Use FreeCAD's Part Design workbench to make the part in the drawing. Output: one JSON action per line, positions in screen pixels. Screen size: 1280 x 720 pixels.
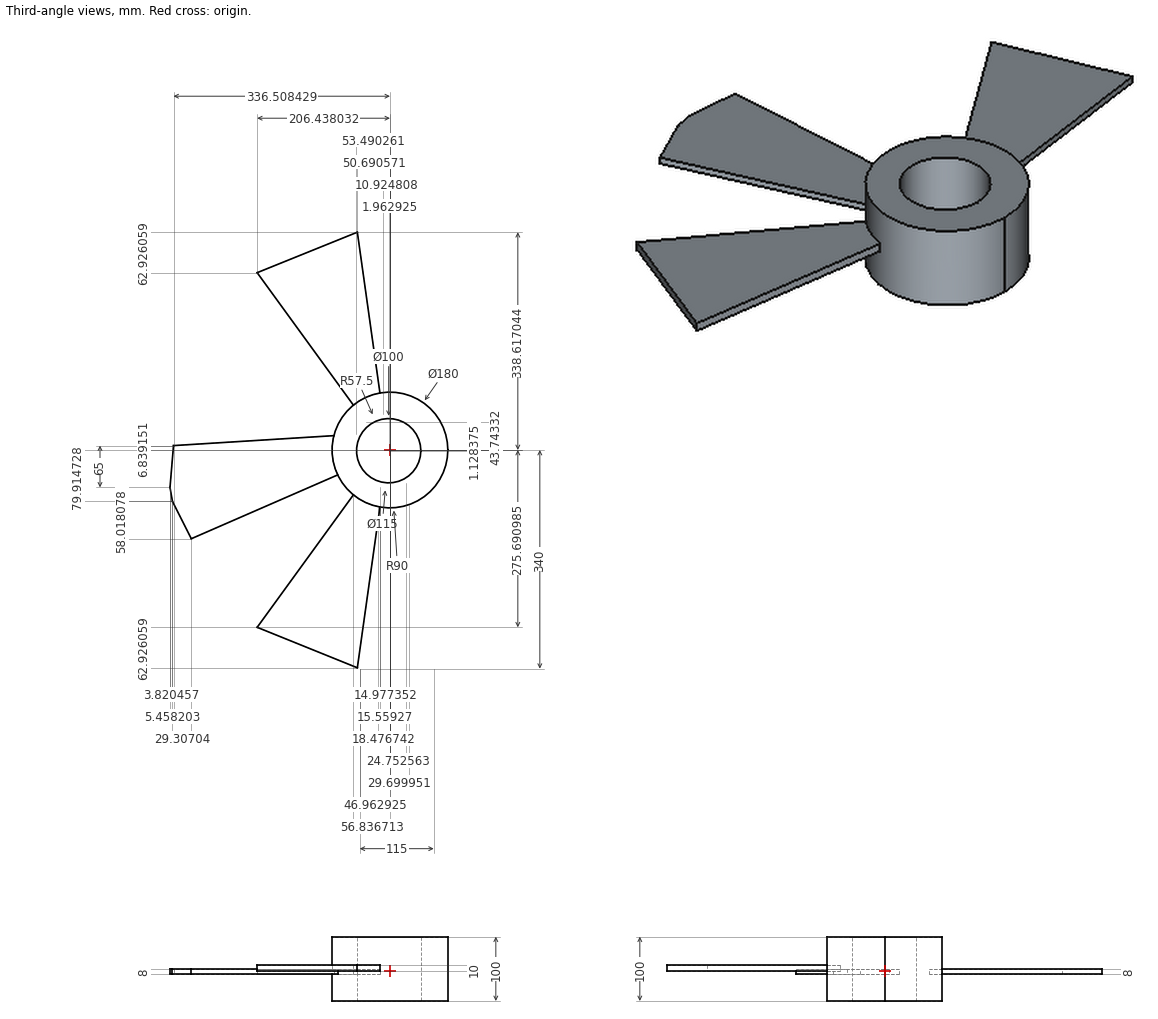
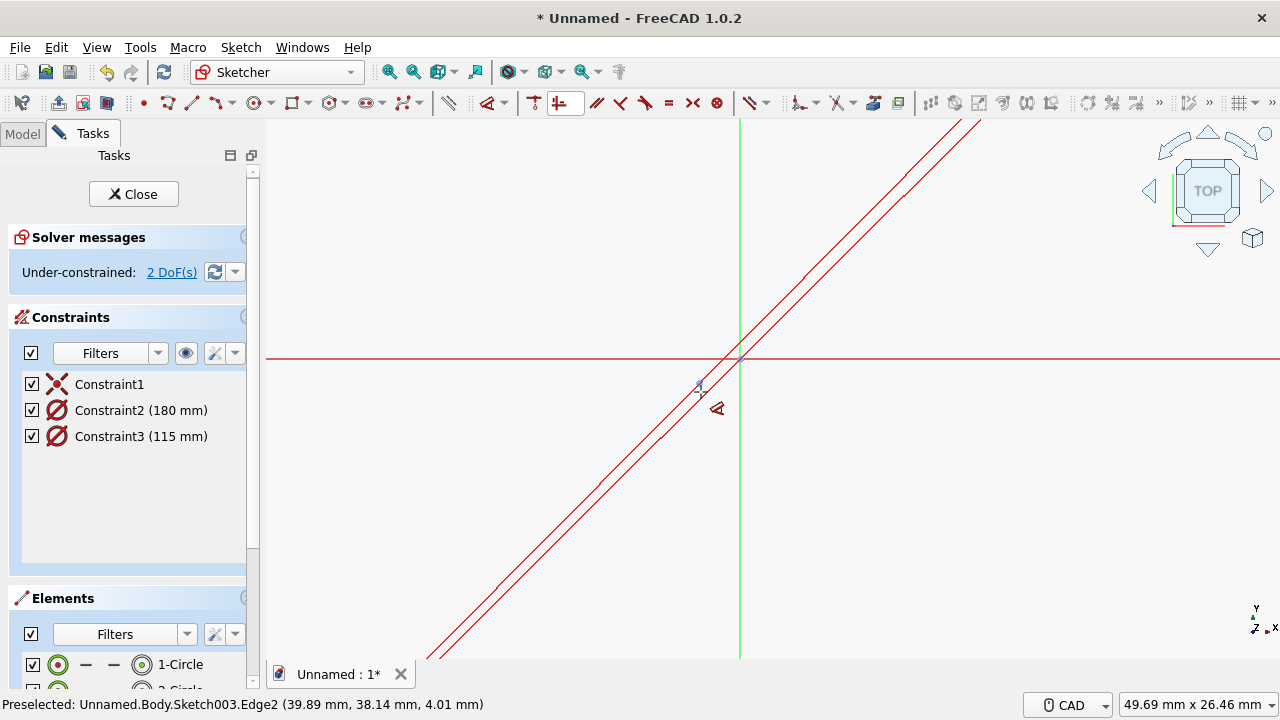
{"action": "left_click", "coordinate": [700, 383]}
{"action": "left_click", "coordinate": [720, 417]}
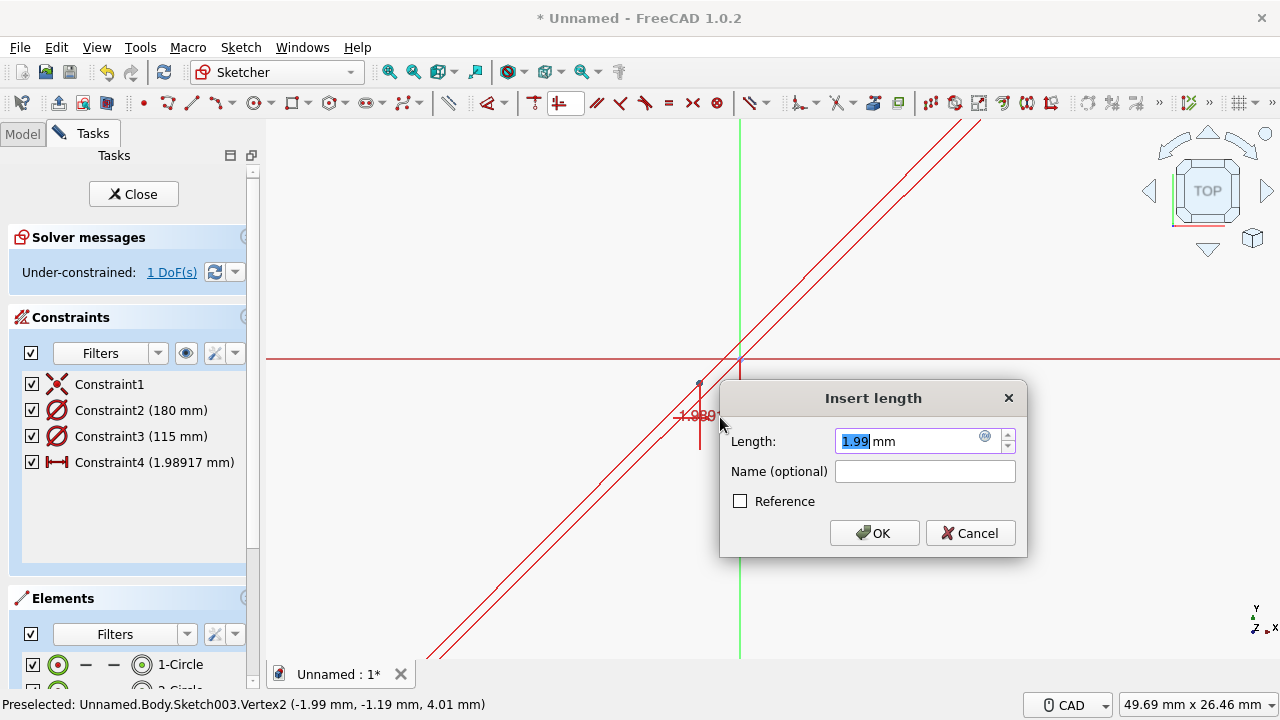
{"action": "type", "text": "1.962925"}
{"action": "key", "text": "Return"}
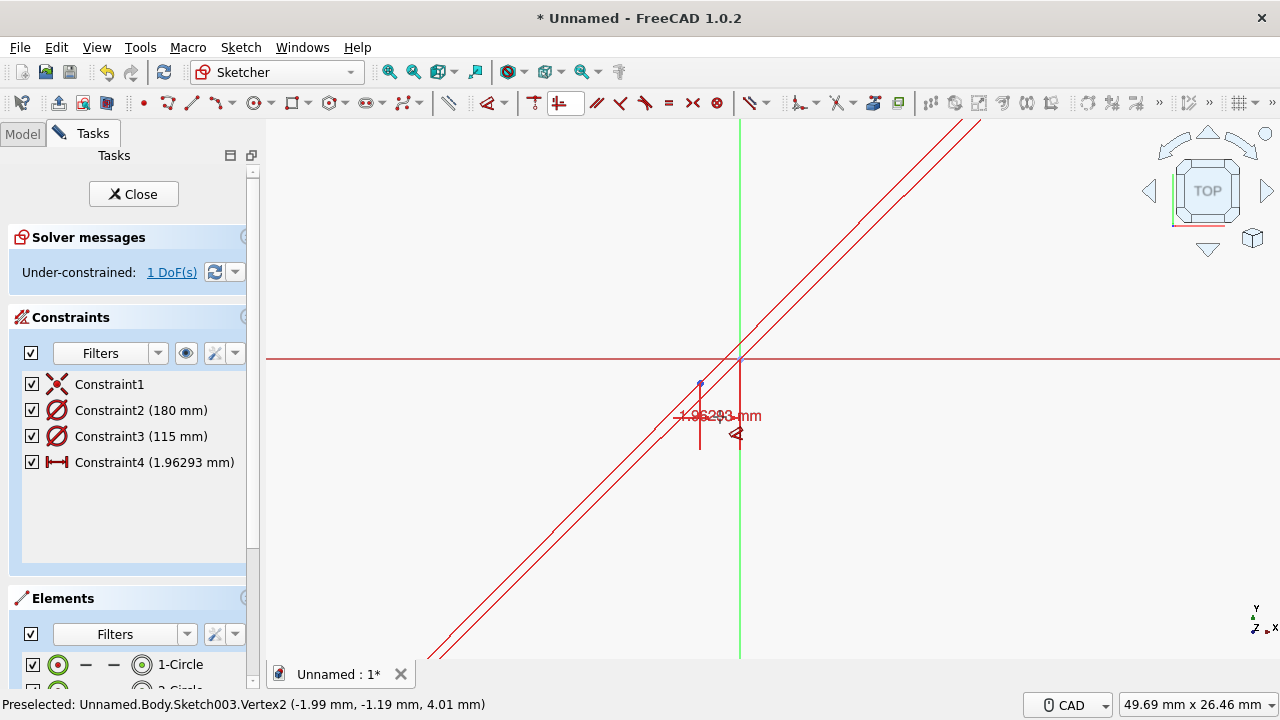
{"action": "scroll", "coordinate": [700, 383], "scroll_direction": "up", "scroll_amount": 3}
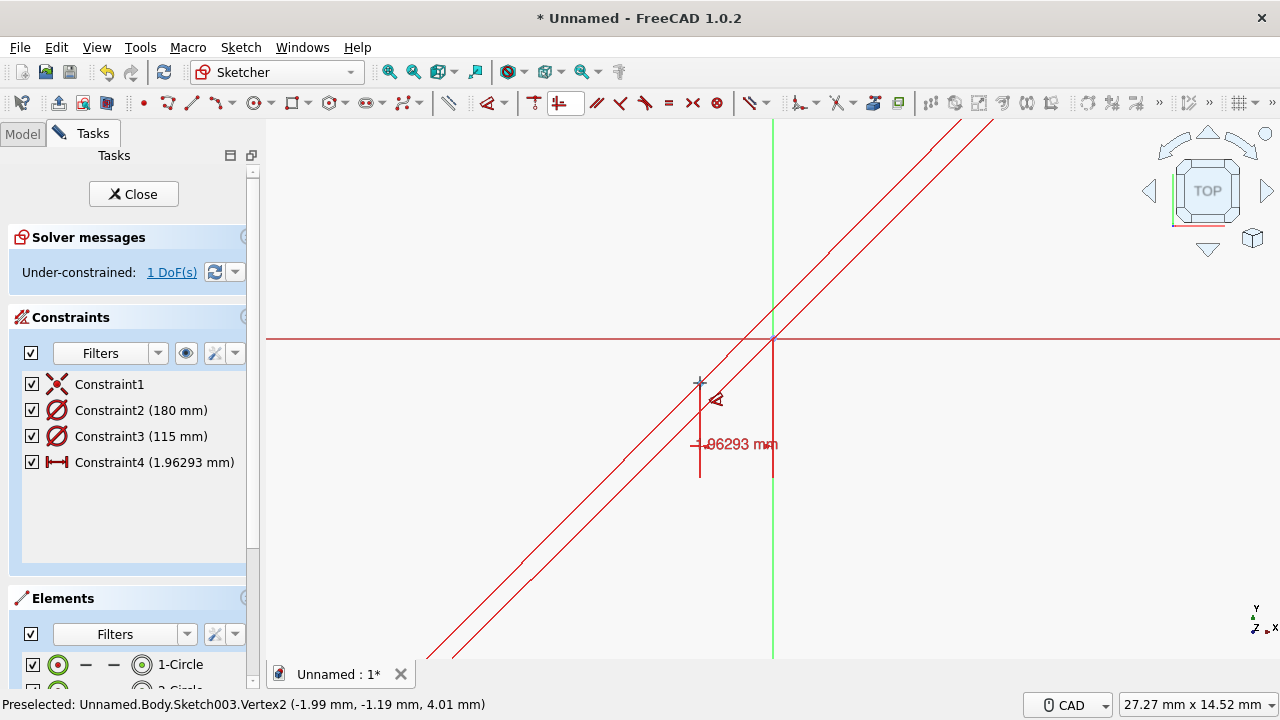
{"action": "left_click", "coordinate": [700, 383]}
{"action": "left_click", "coordinate": [666, 361]}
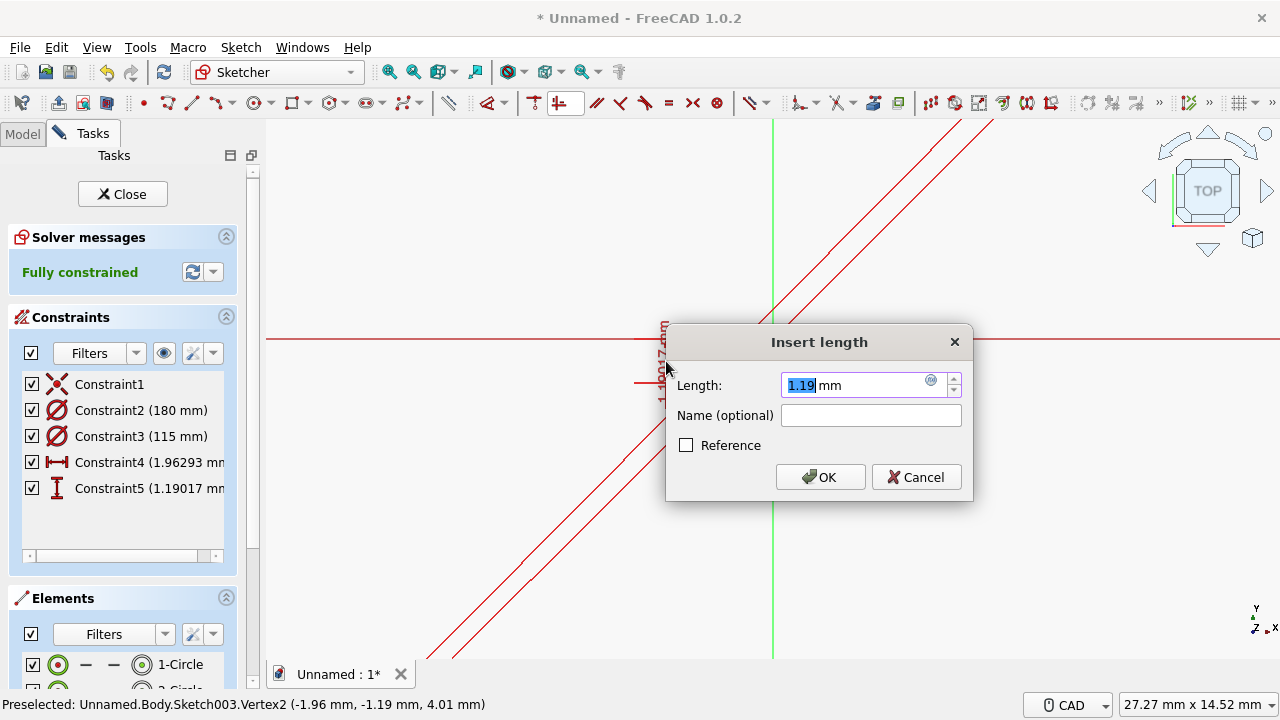
{"action": "type", "text": "1.128375"}
{"action": "key", "text": "Return"}
{"action": "key", "text": "Escape"}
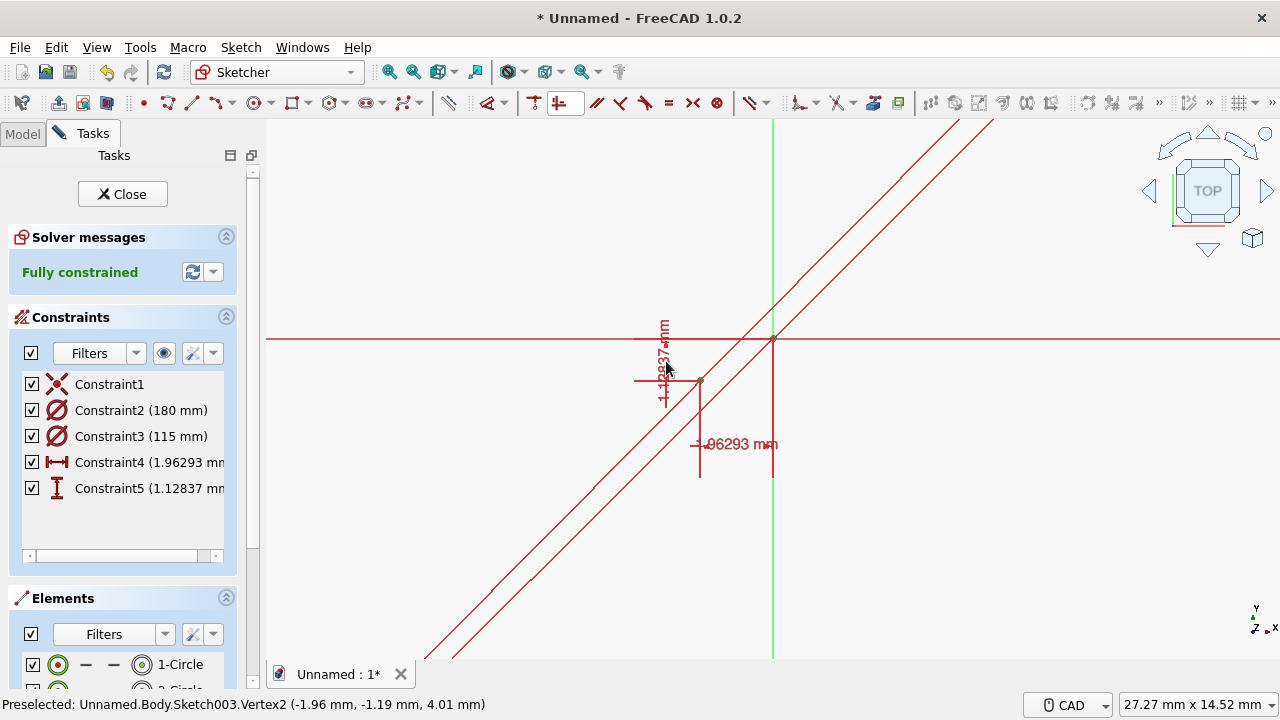
{"action": "left_click", "coordinate": [123, 194]}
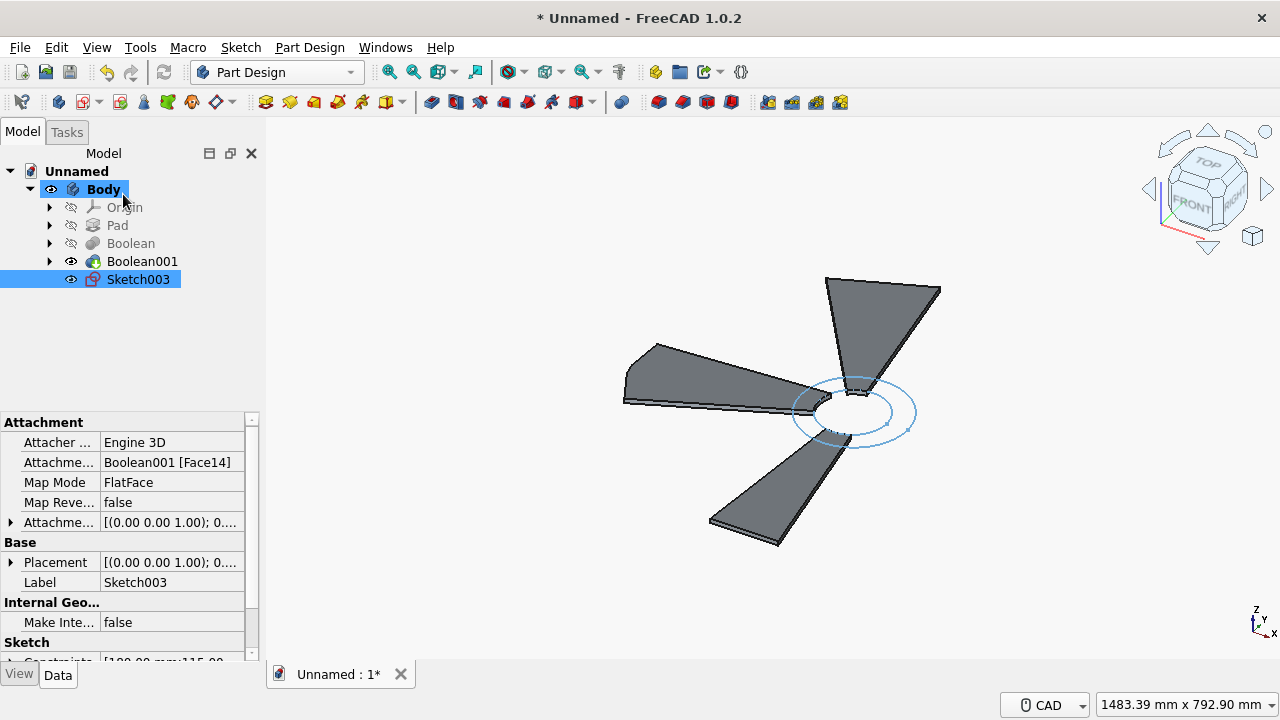
{"action": "left_click", "coordinate": [266, 102]}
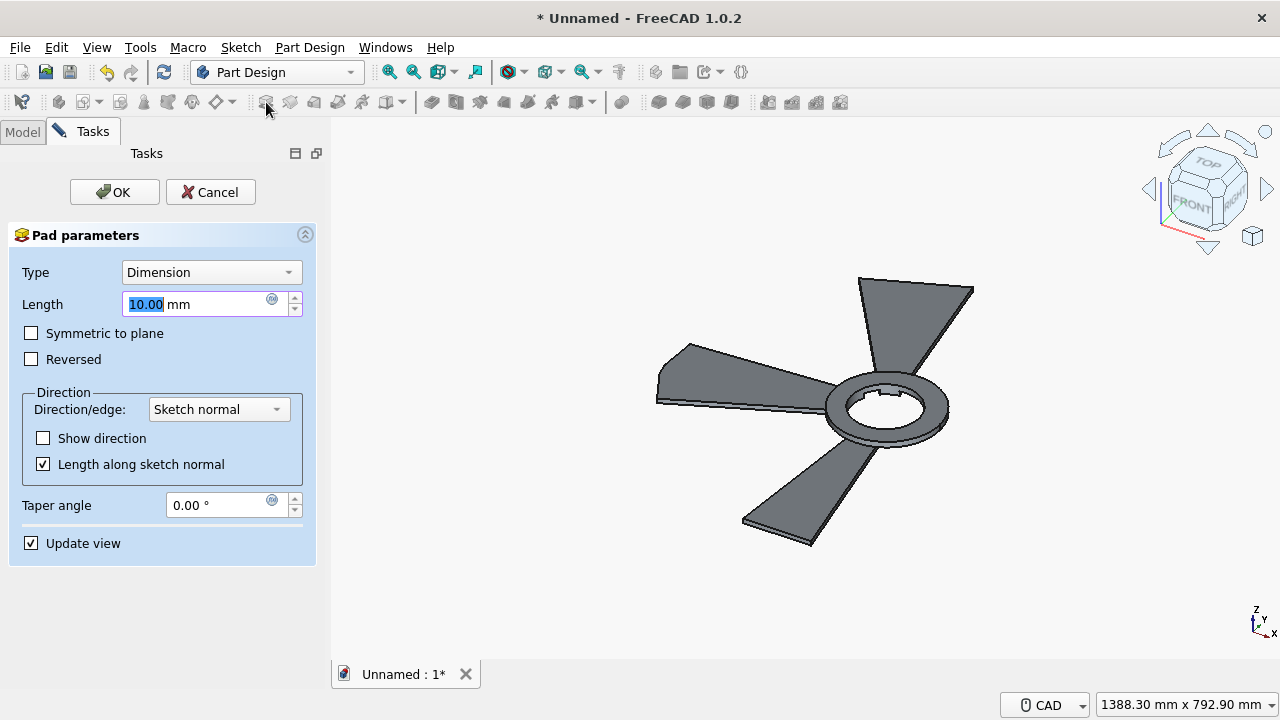
{"action": "type", "text": "100"}
{"action": "key", "text": "Tab"}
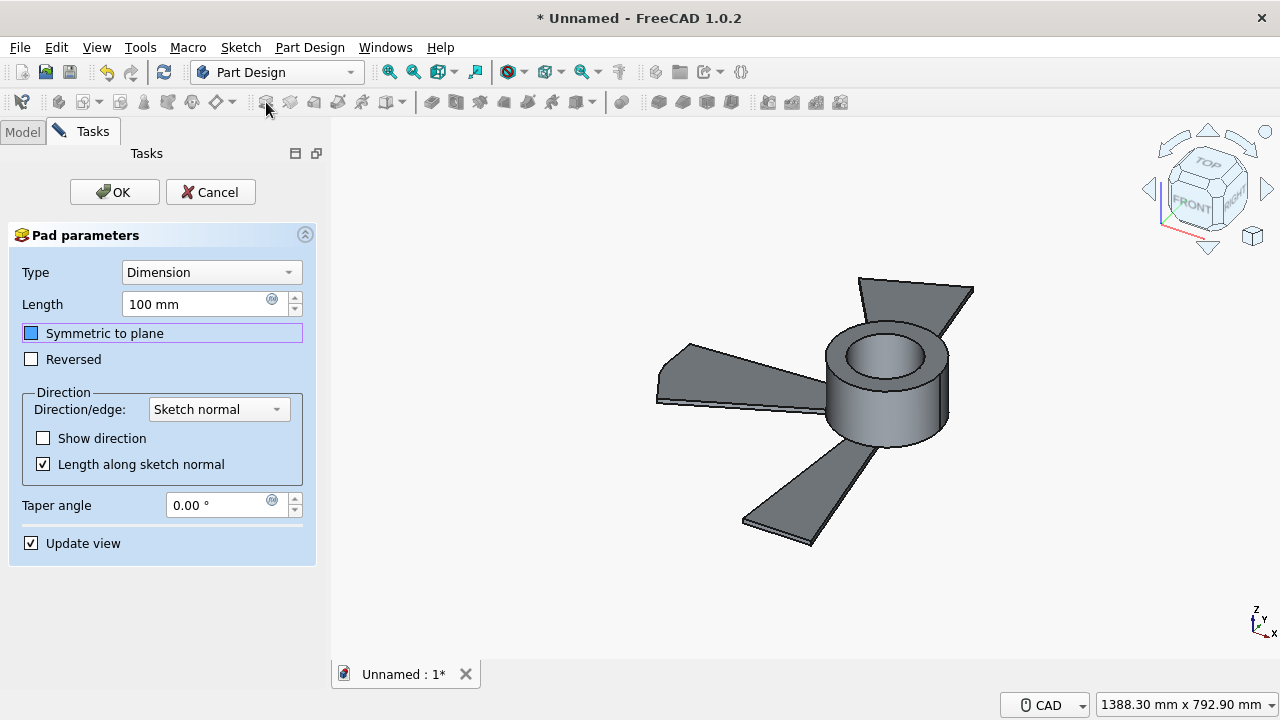
{"action": "left_click", "coordinate": [30, 333]}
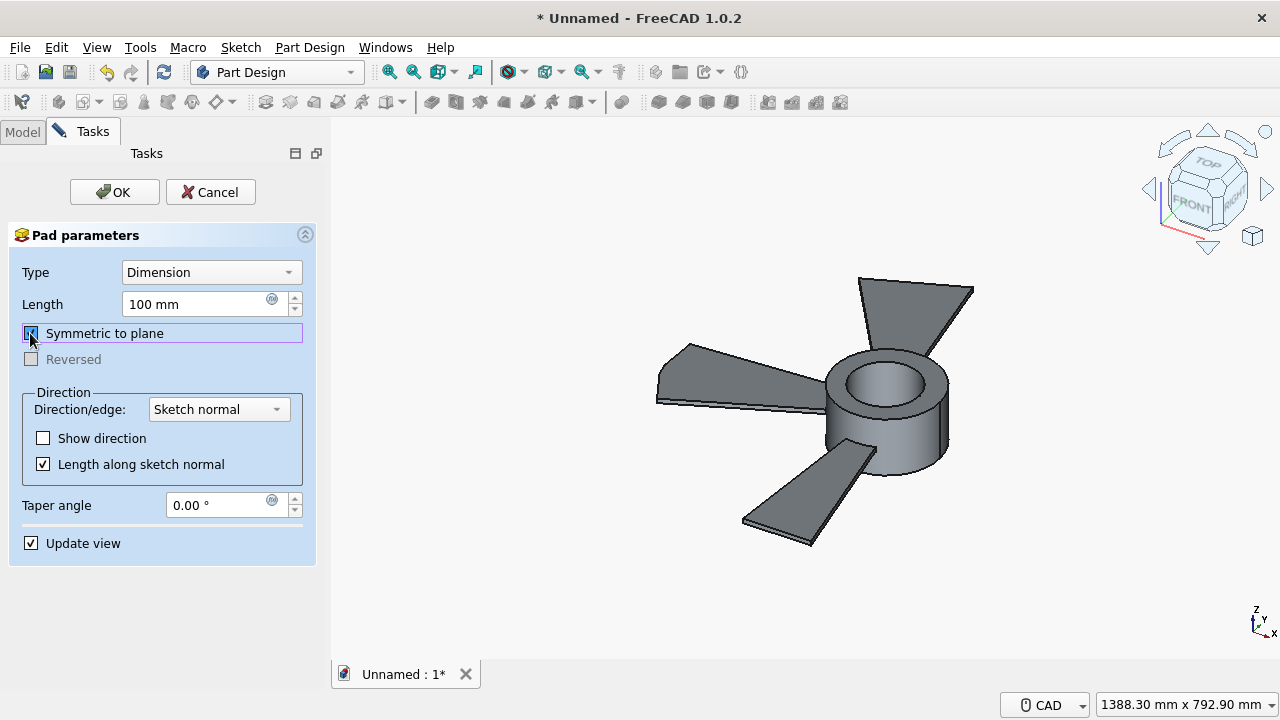
{"action": "left_click", "coordinate": [115, 192]}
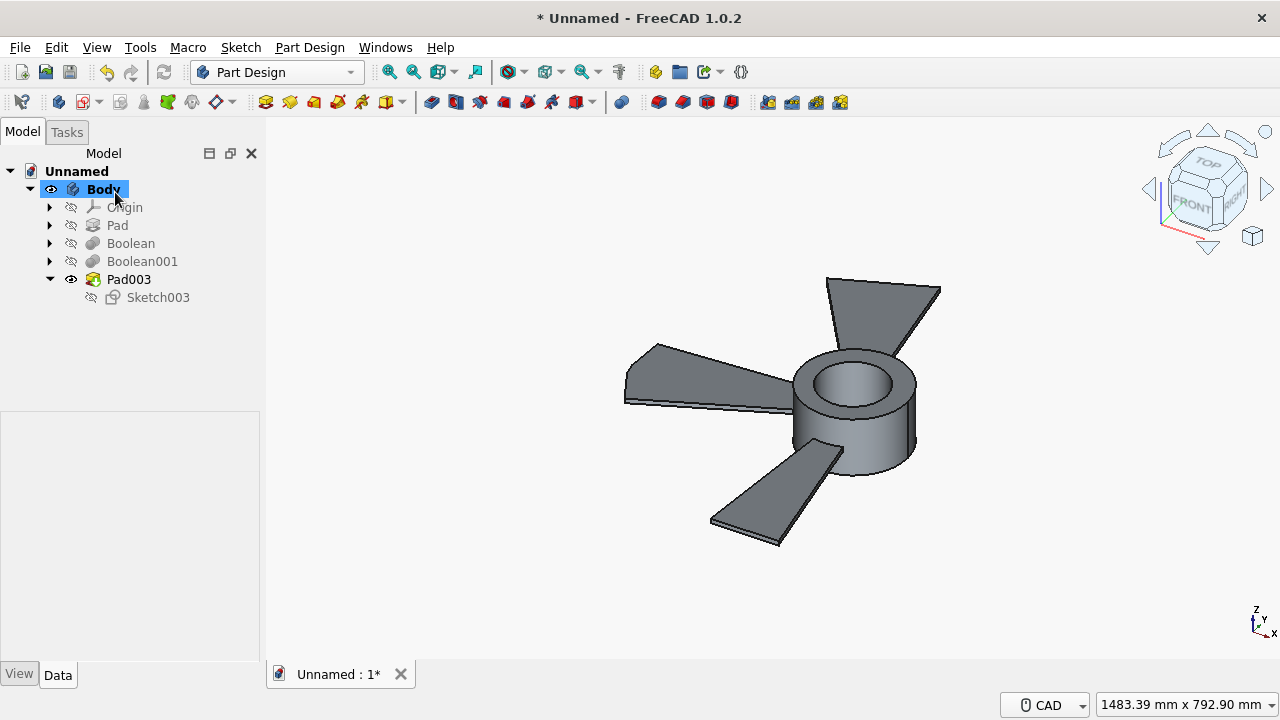
{"action": "left_click", "coordinate": [903, 376]}